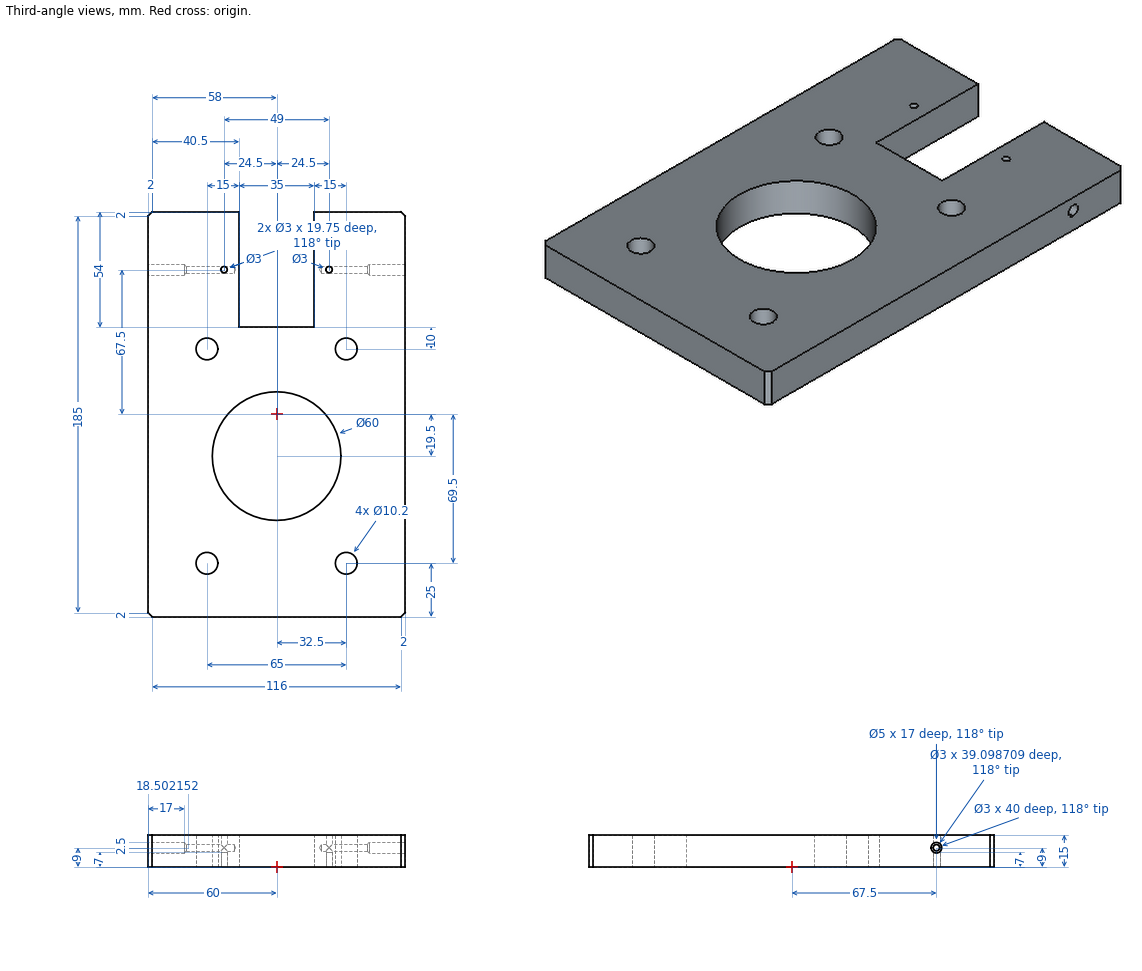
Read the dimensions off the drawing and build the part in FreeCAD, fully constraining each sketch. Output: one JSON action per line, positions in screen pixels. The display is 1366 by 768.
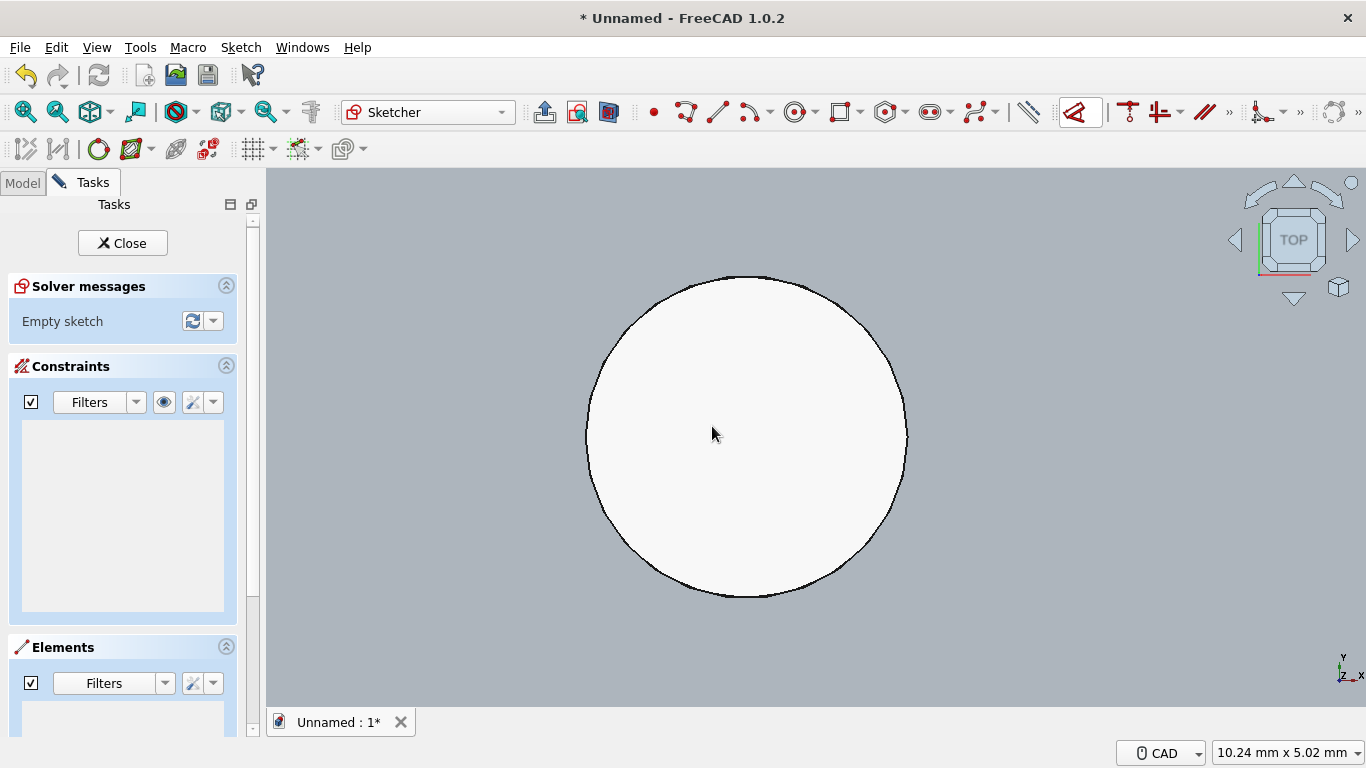
{"action": "left_click", "coordinate": [796, 112]}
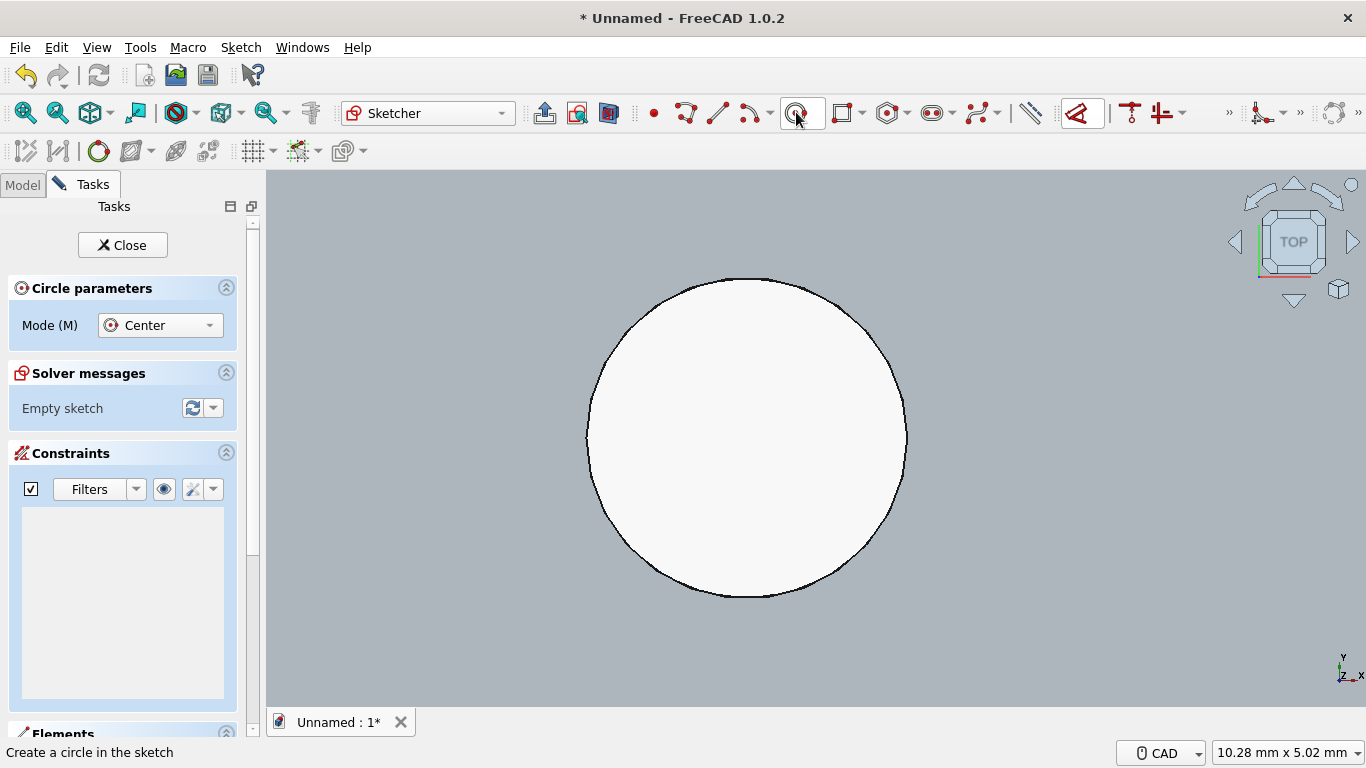
{"action": "left_click", "coordinate": [747, 438]}
{"action": "mouse_move", "coordinate": [860, 325]}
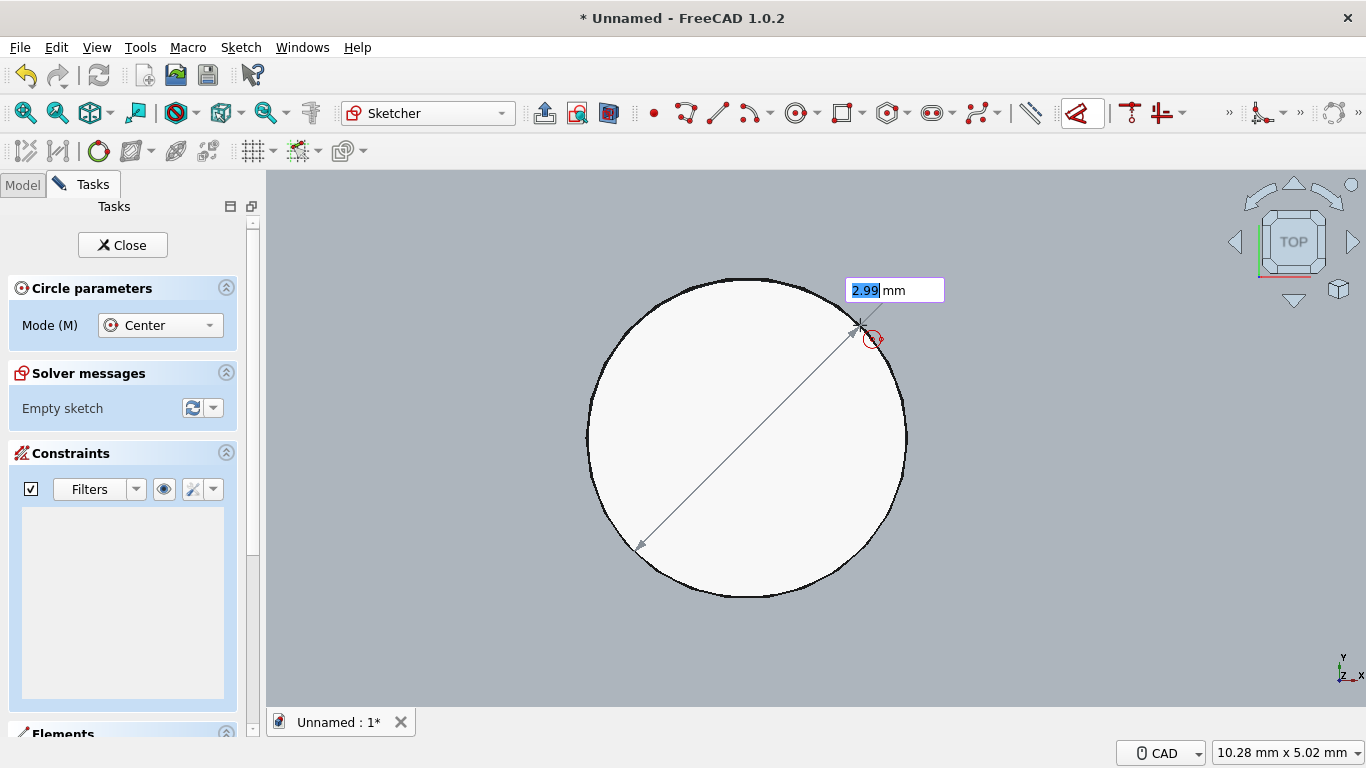
{"action": "type", "text": "3"}
{"action": "key", "text": "Return"}
{"action": "key", "text": "Escape"}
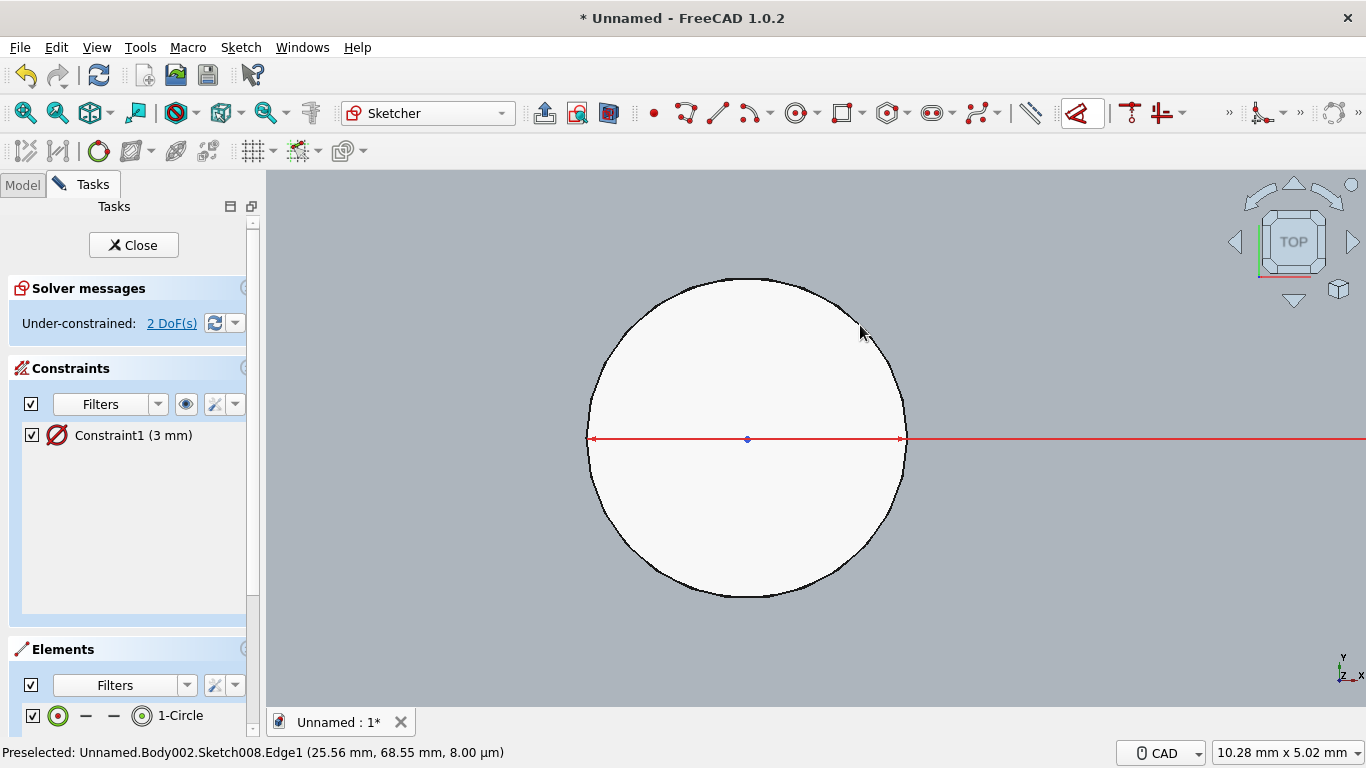
{"action": "left_click", "coordinate": [747, 439]}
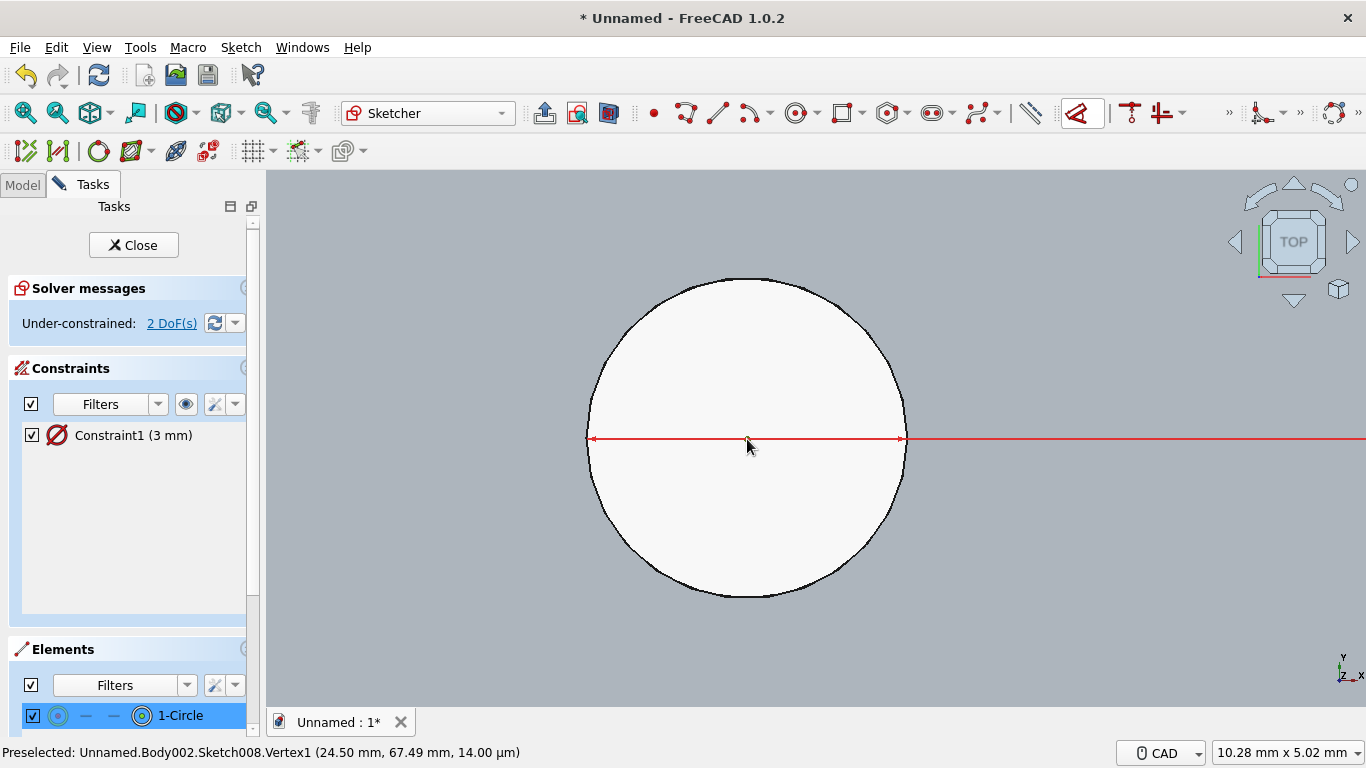
{"action": "left_click", "coordinate": [1098, 114]}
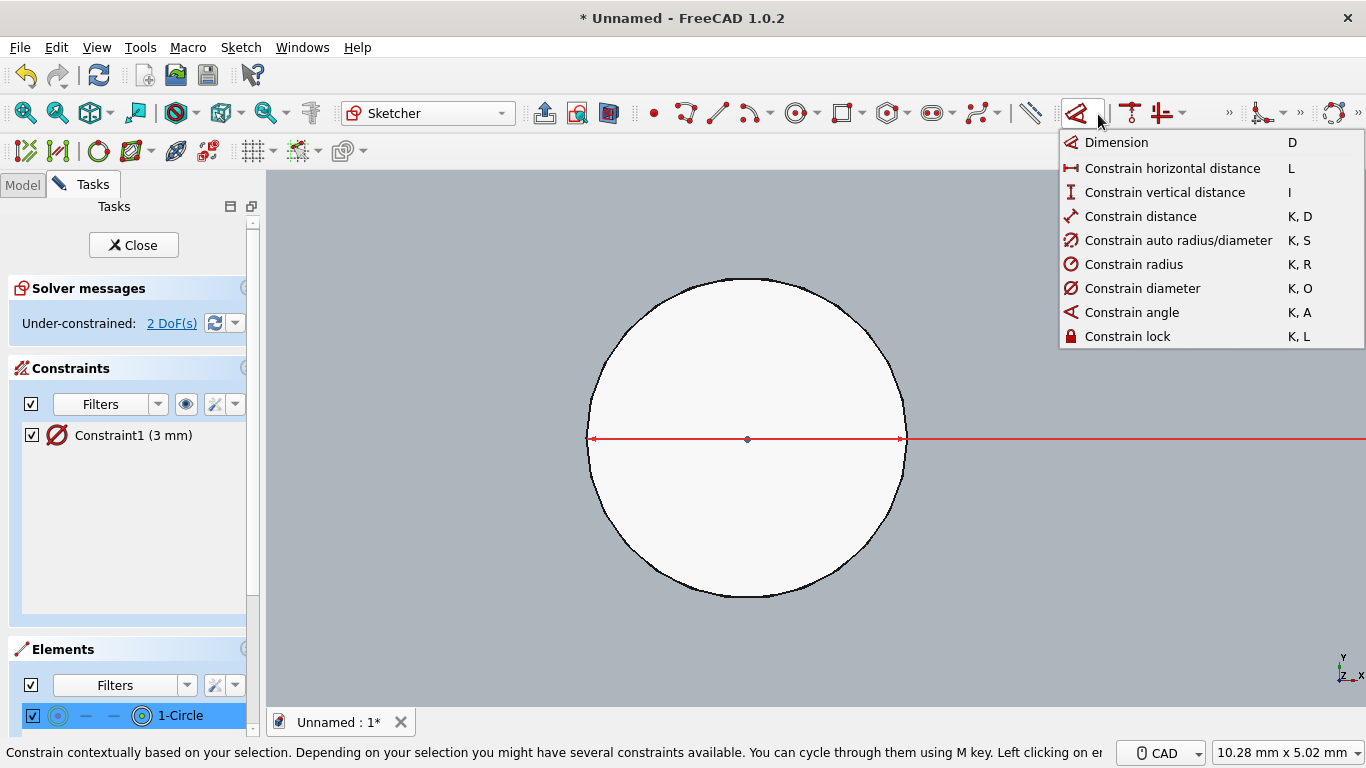
{"action": "left_click", "coordinate": [1212, 168]}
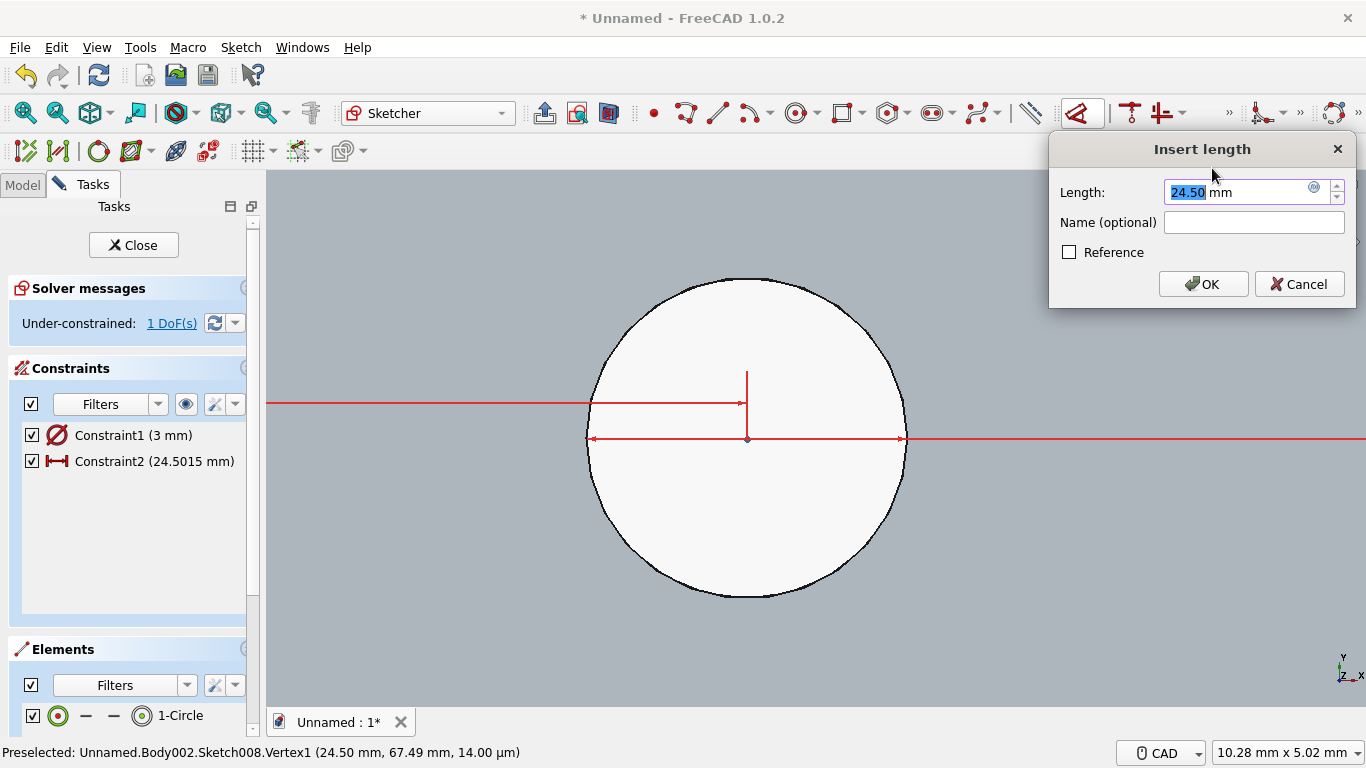
{"action": "type", "text": "24.5"}
{"action": "key", "text": "Return"}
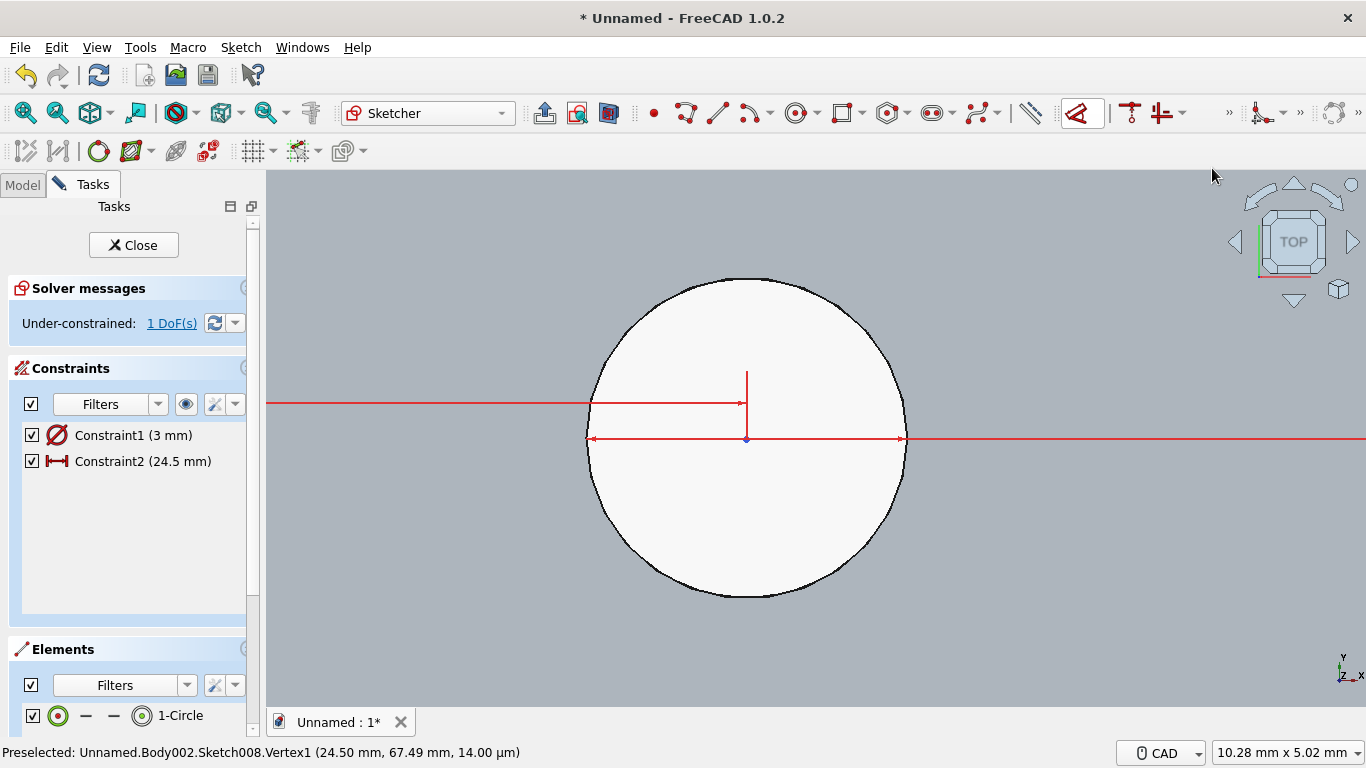
{"action": "left_click", "coordinate": [747, 439]}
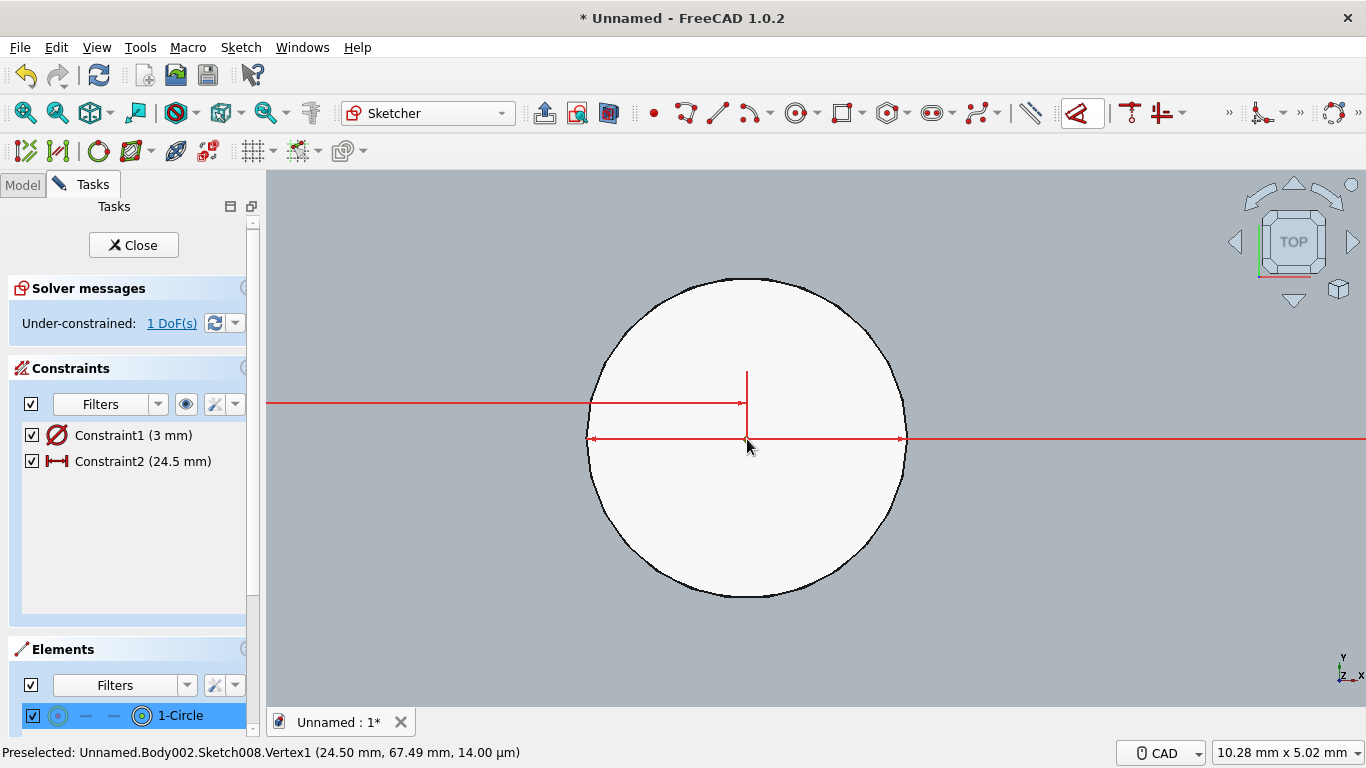
{"action": "key", "text": "i"}